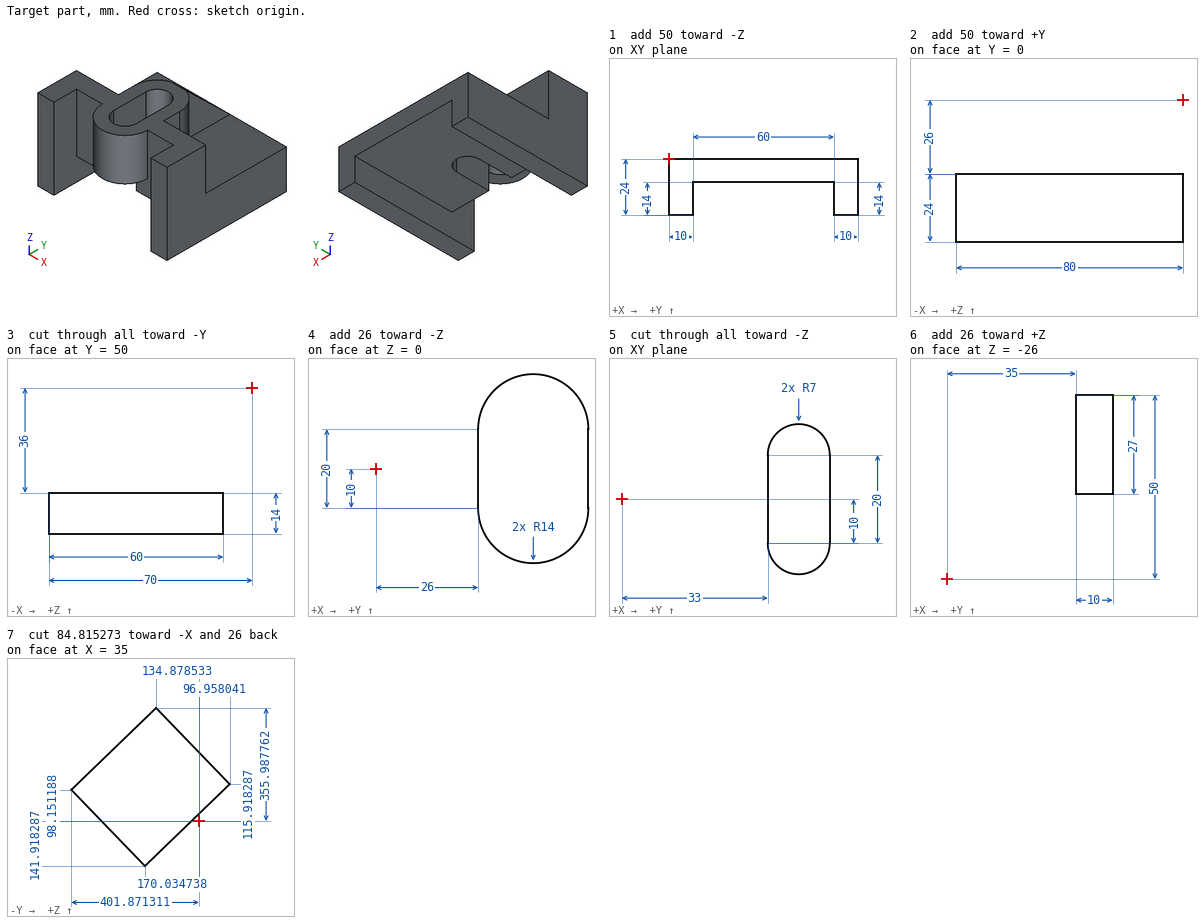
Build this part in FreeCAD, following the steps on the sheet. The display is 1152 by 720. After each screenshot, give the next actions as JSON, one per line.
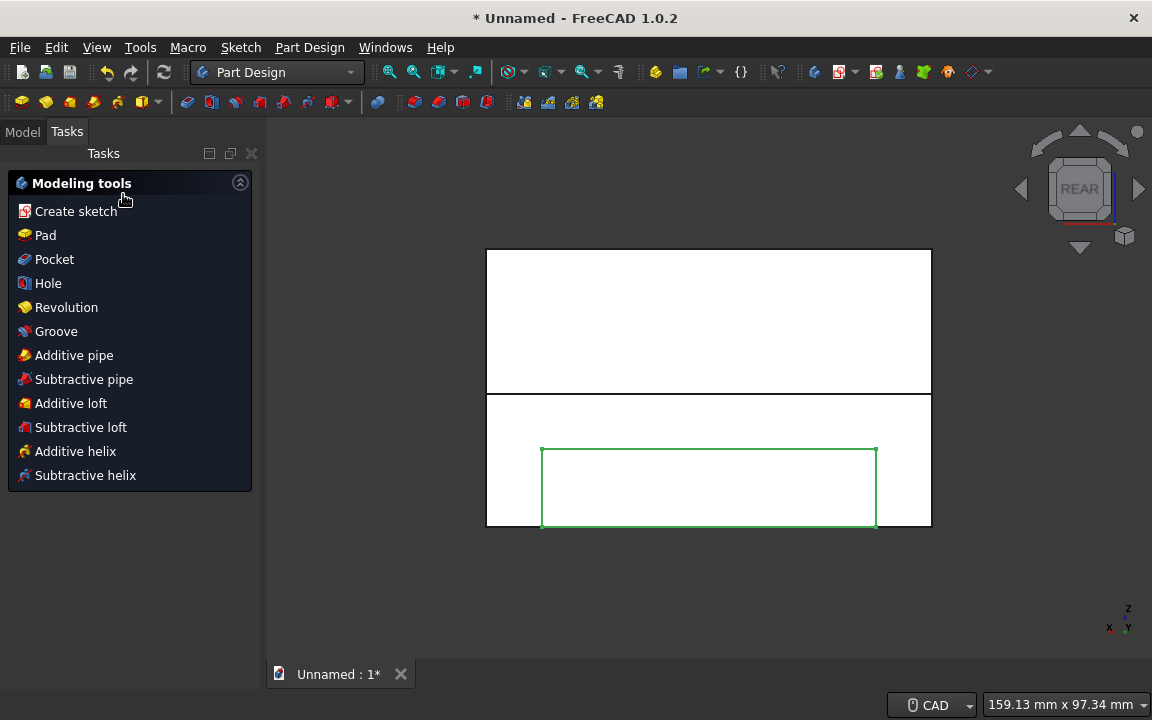
{"action": "left_click", "coordinate": [188, 102]}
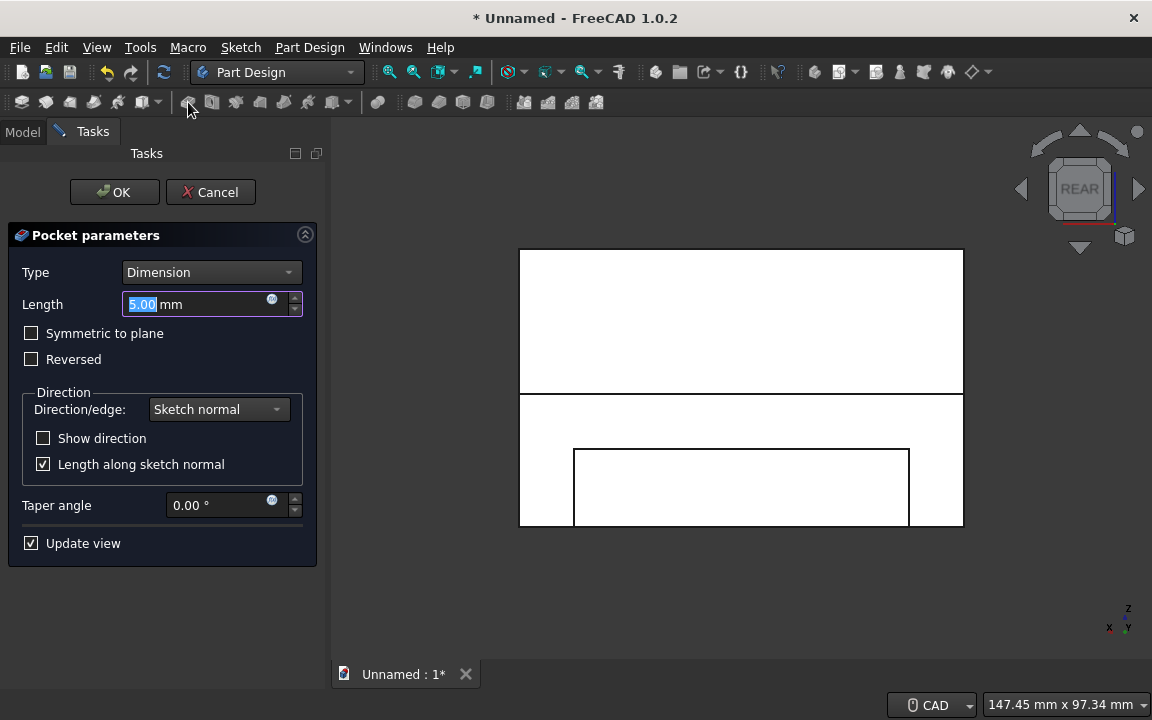
{"action": "left_click", "coordinate": [212, 272]}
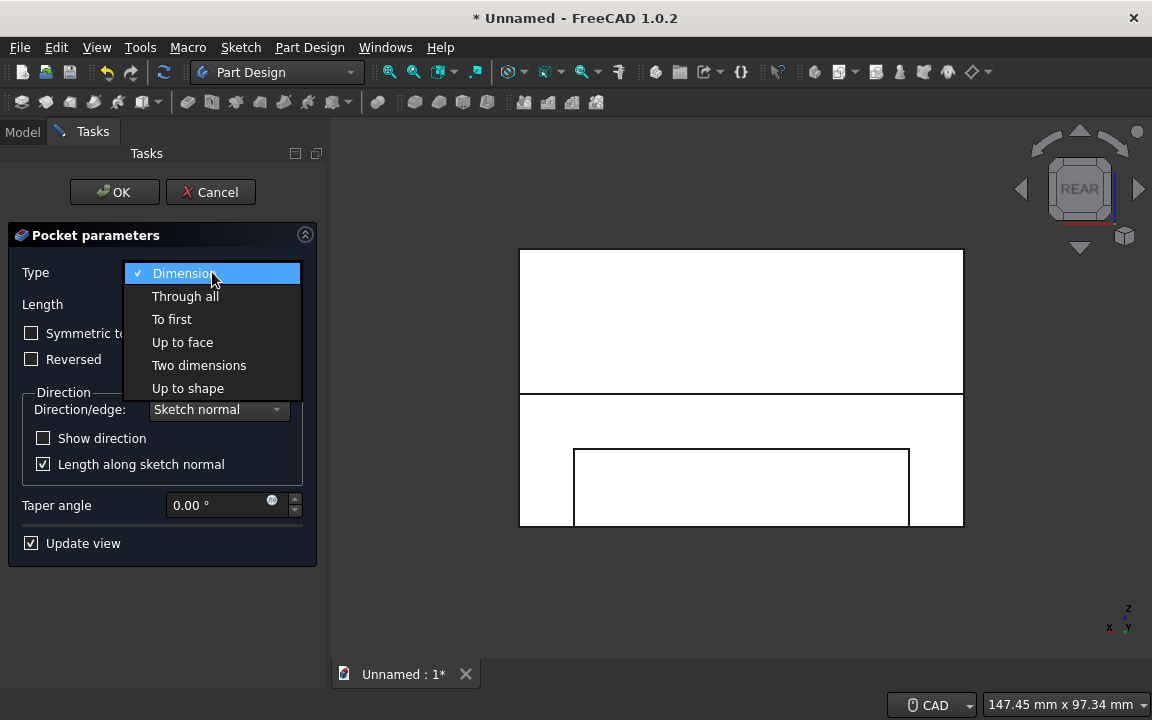
{"action": "left_click", "coordinate": [212, 296]}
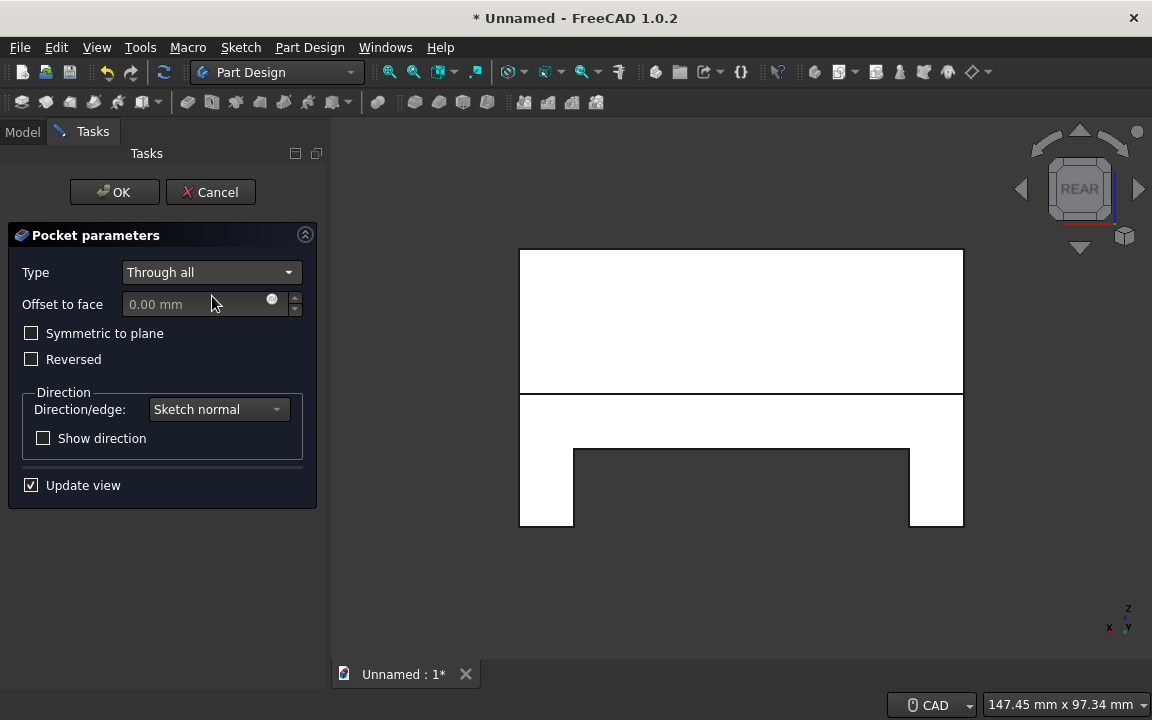
{"action": "left_click", "coordinate": [115, 192]}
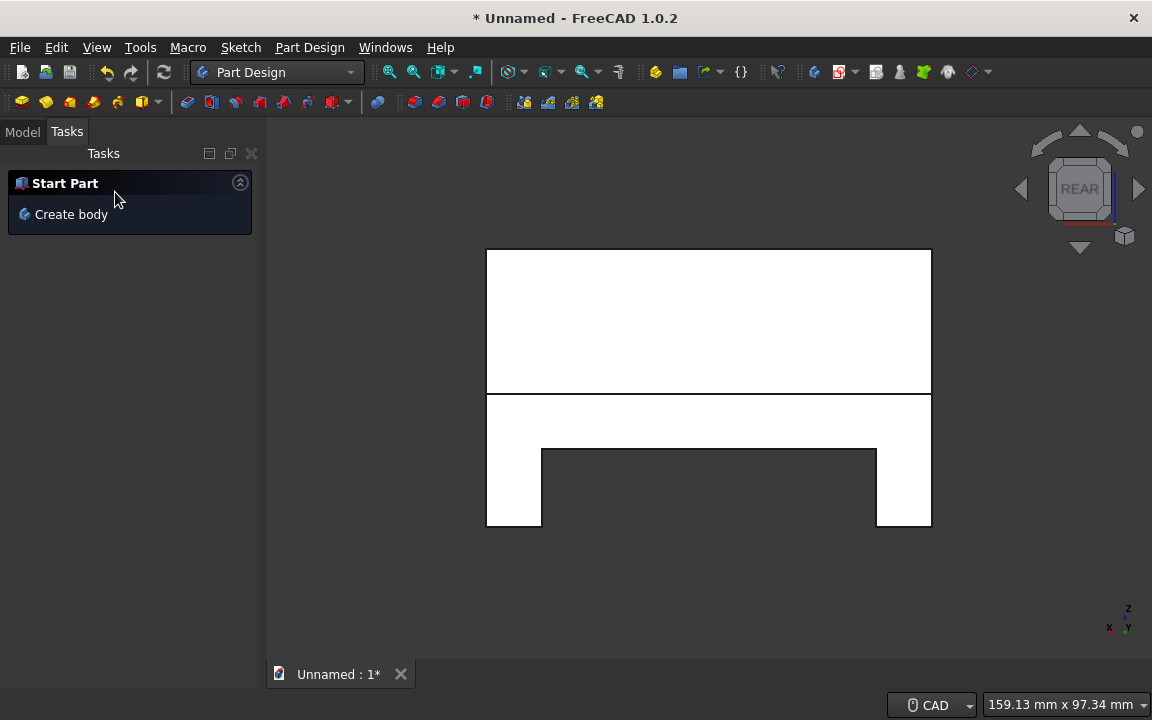
{"action": "key", "text": "0"}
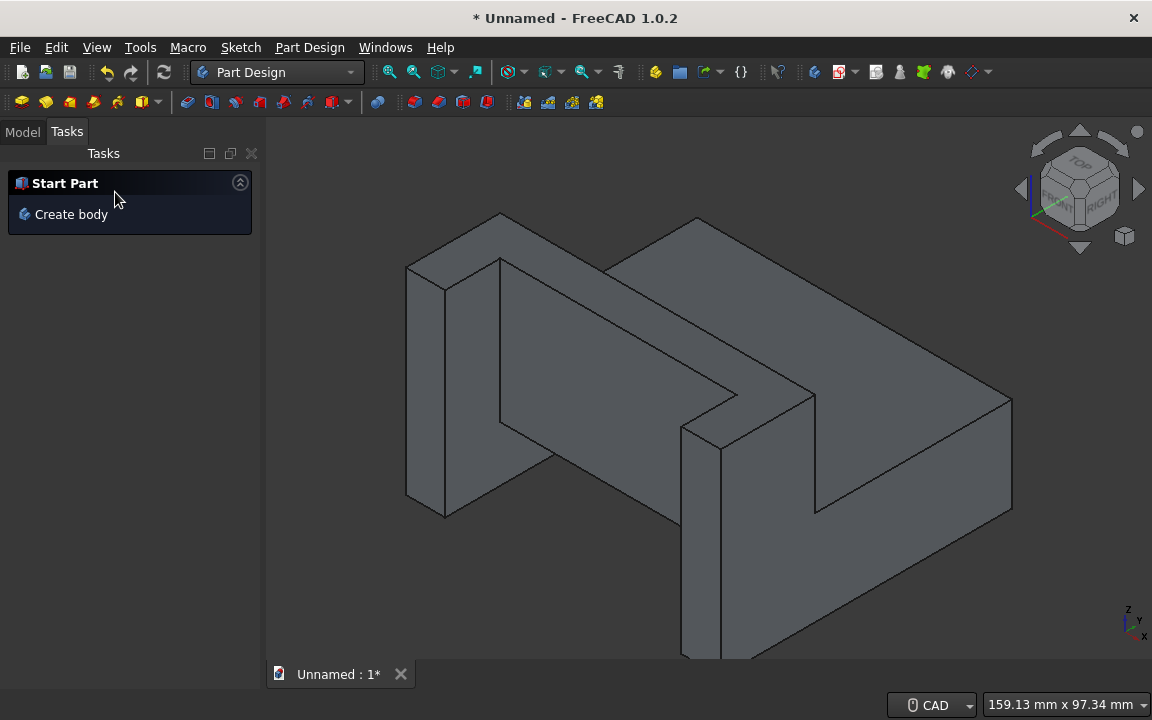
{"action": "key", "text": "v f"}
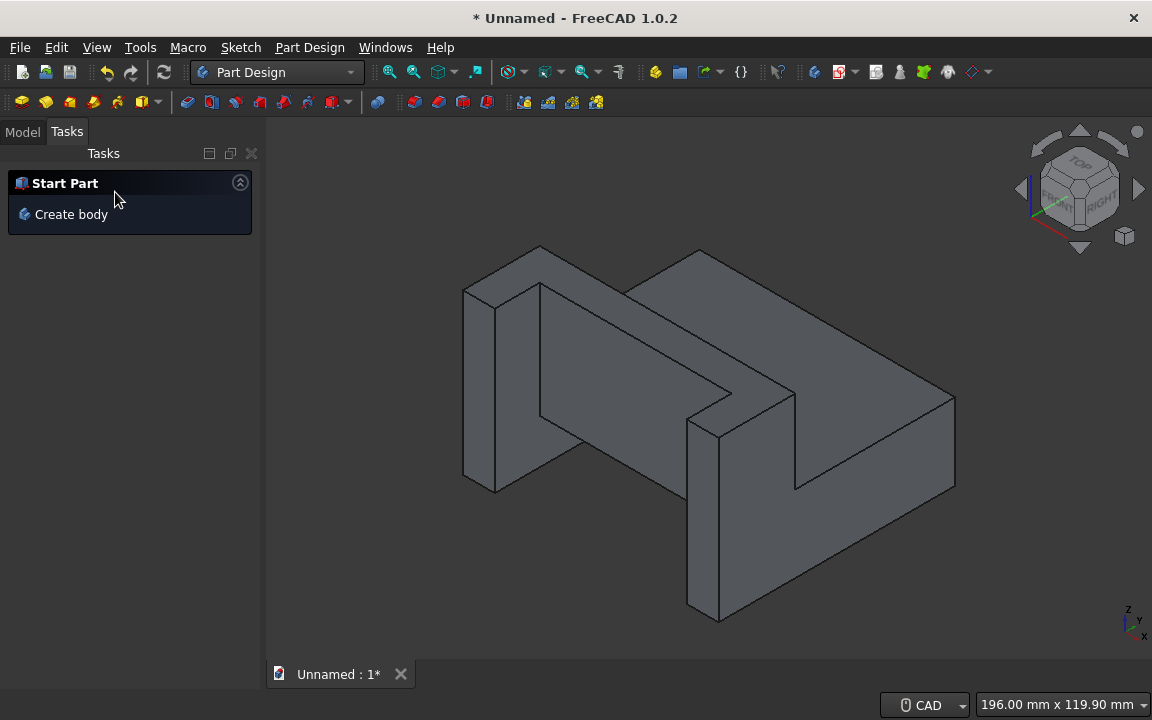
{"action": "left_click", "coordinate": [761, 391]}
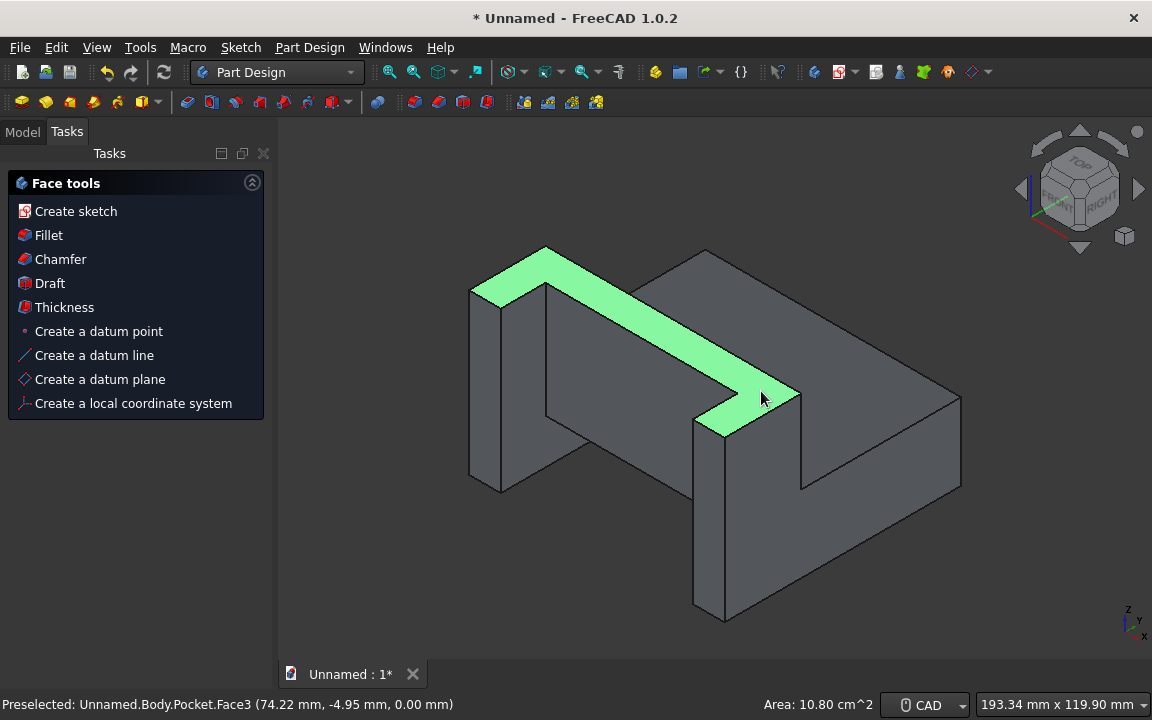
{"action": "left_click", "coordinate": [840, 72]}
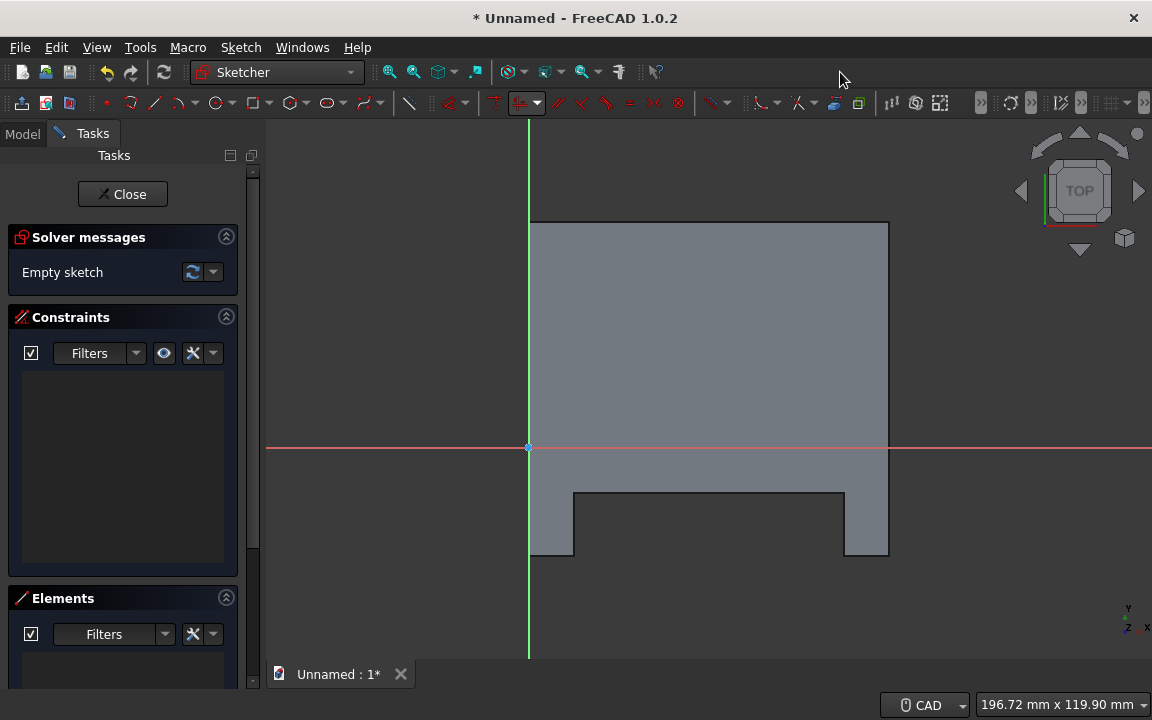
{"action": "scroll", "coordinate": [671, 567], "scroll_direction": "up", "scroll_amount": 2}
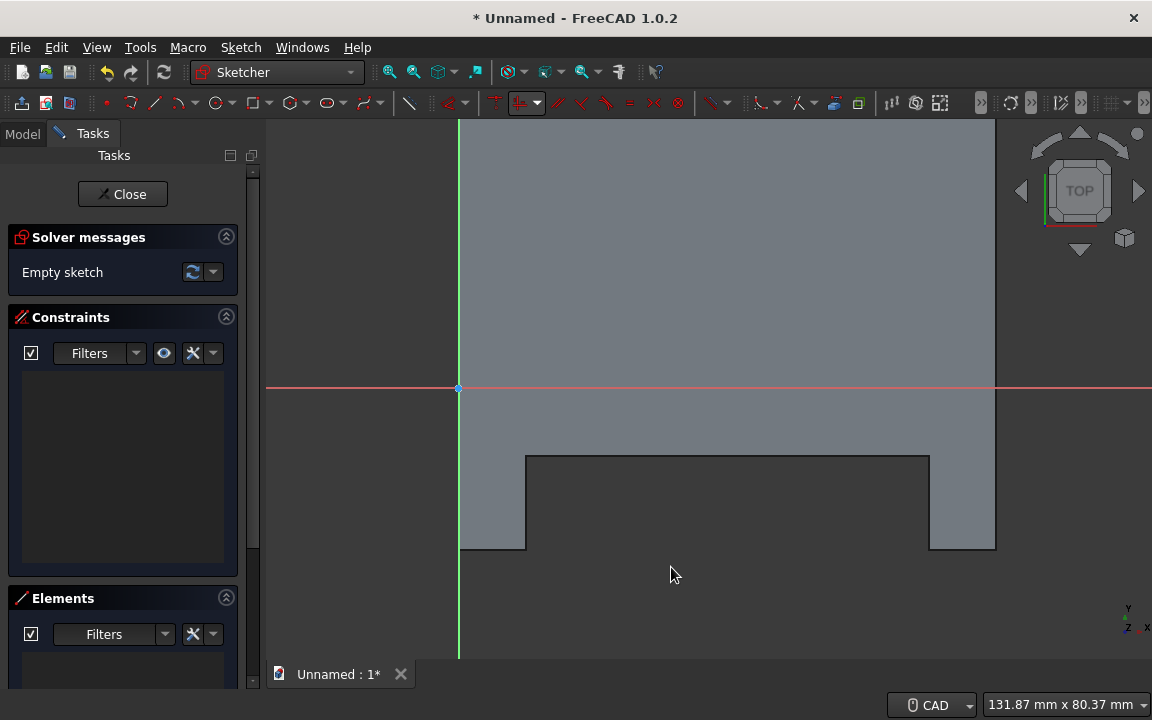
{"action": "key", "text": "g s"}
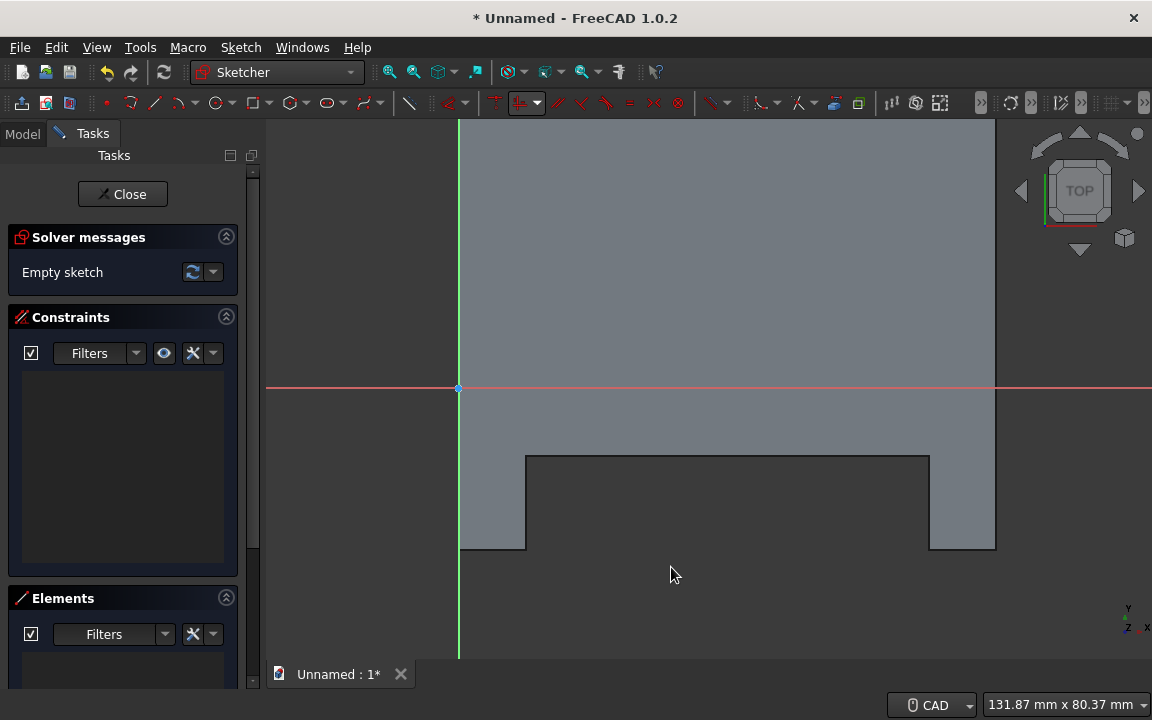
{"action": "left_click", "coordinate": [727, 456]}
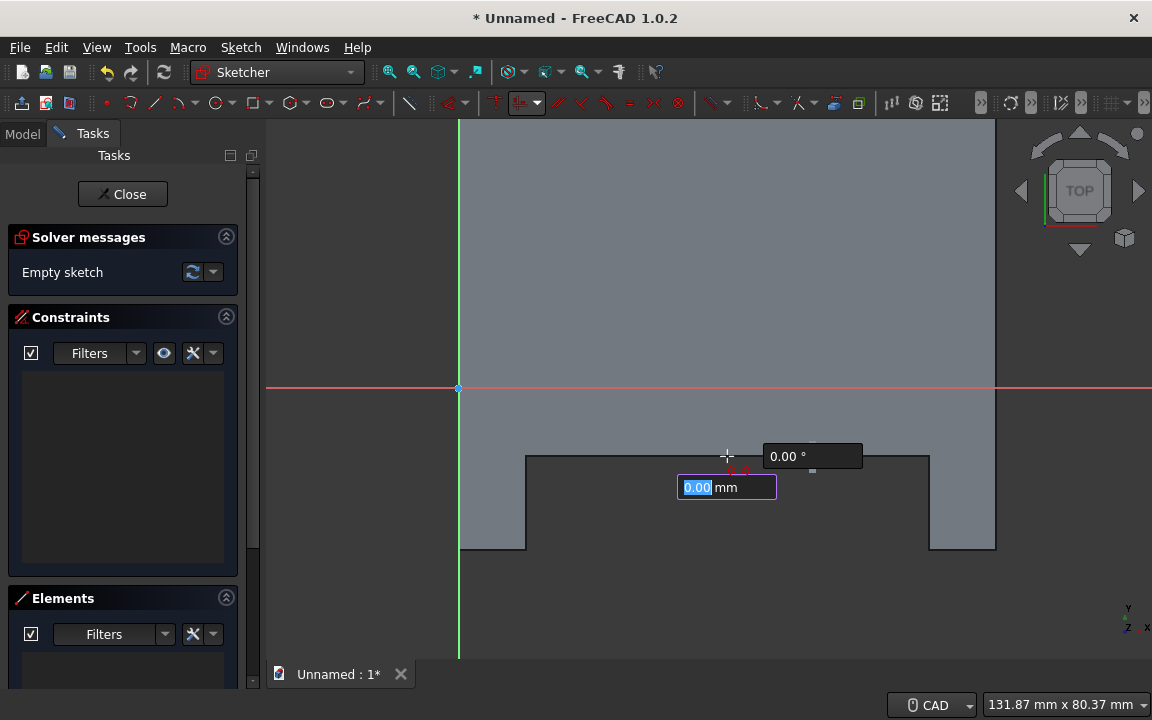
{"action": "left_click", "coordinate": [727, 321]}